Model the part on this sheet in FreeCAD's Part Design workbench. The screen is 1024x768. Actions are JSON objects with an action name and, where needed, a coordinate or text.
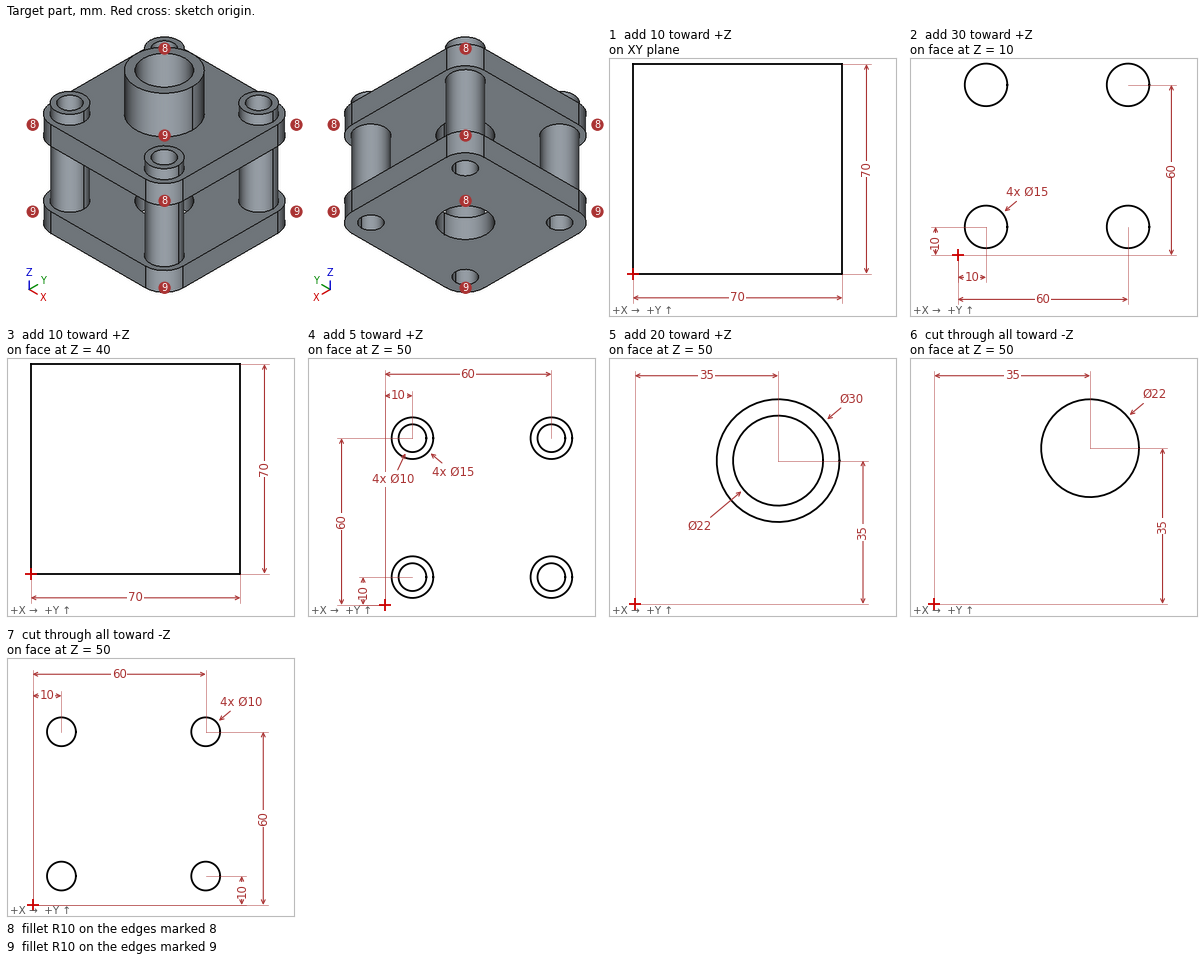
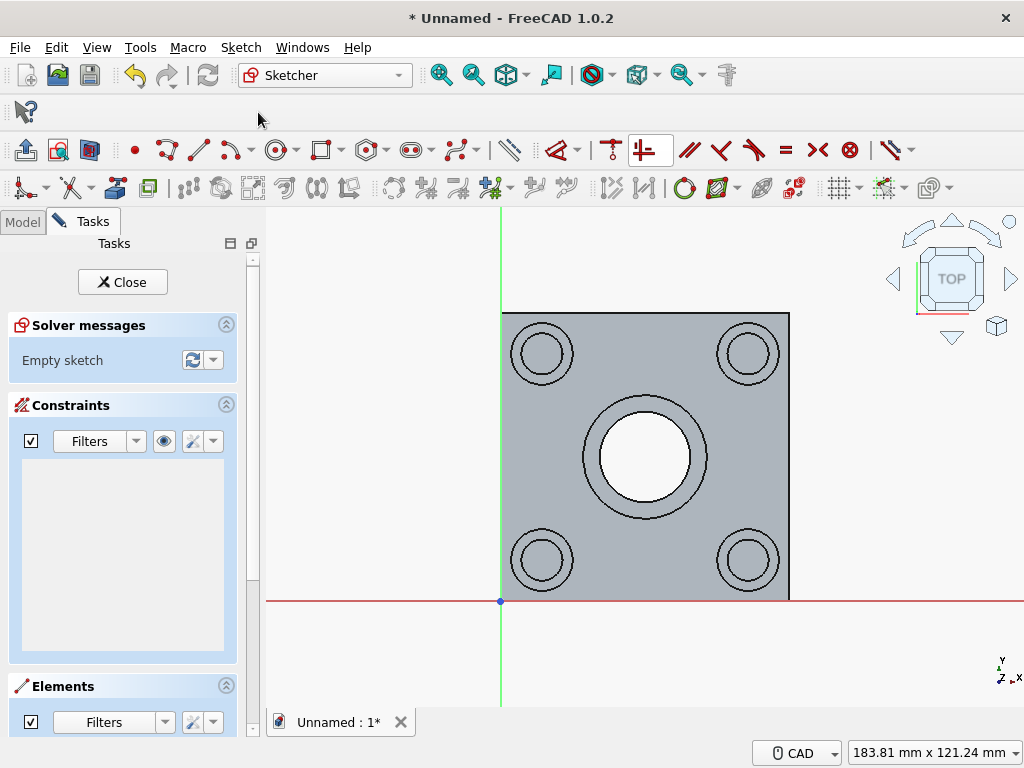
{"action": "left_click", "coordinate": [276, 150]}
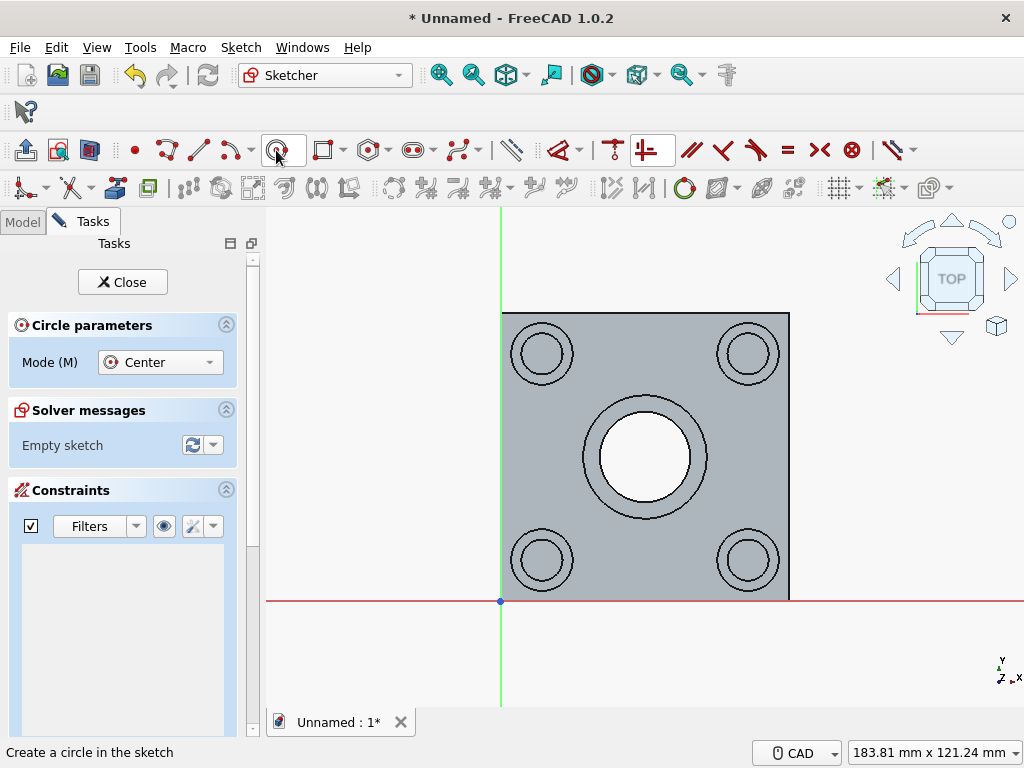
{"action": "left_click", "coordinate": [748, 354]}
{"action": "left_click", "coordinate": [763, 339]}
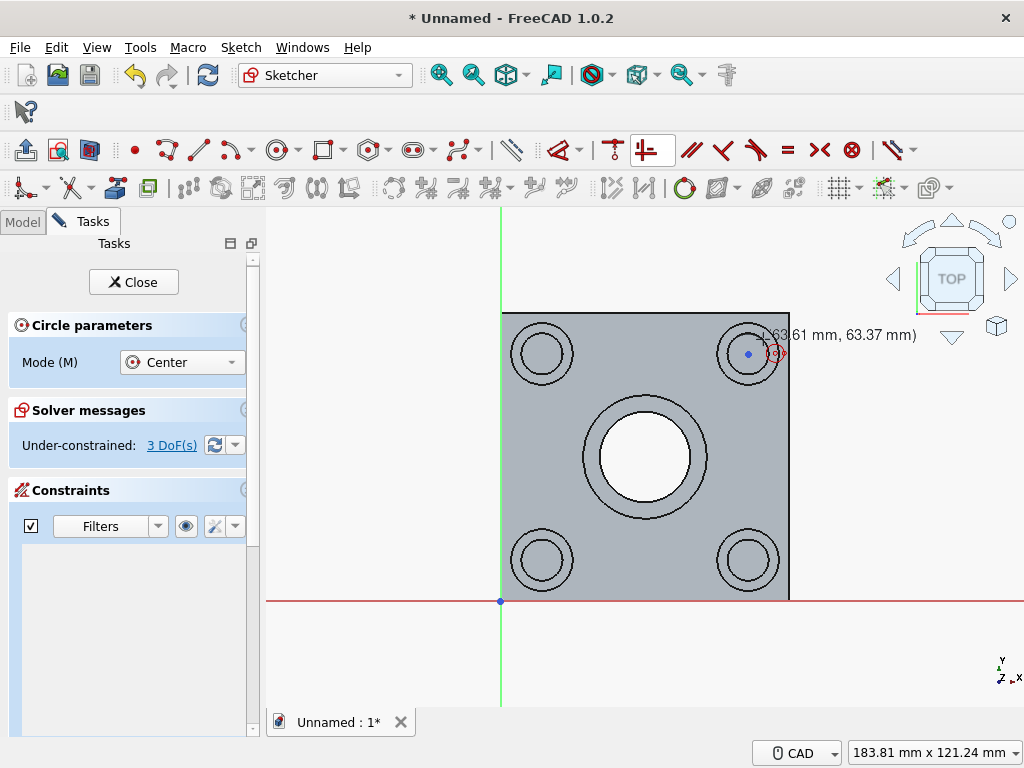
{"action": "left_click", "coordinate": [542, 354]}
{"action": "left_click", "coordinate": [556, 339]}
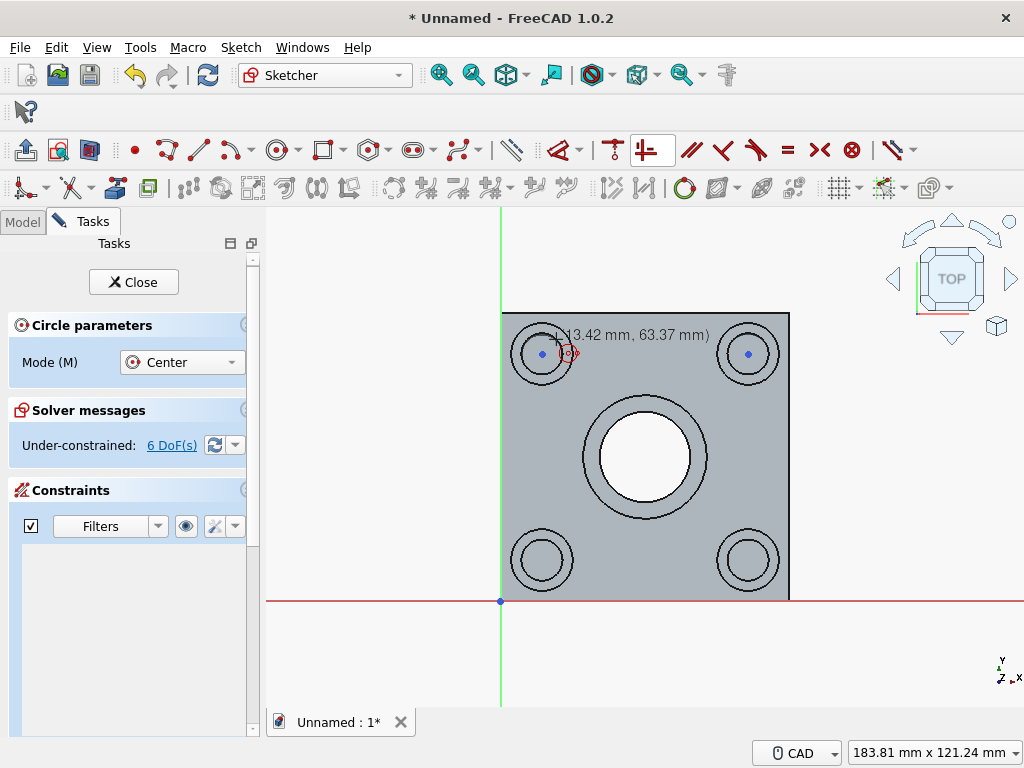
{"action": "left_click", "coordinate": [748, 560]}
{"action": "left_click", "coordinate": [763, 546]}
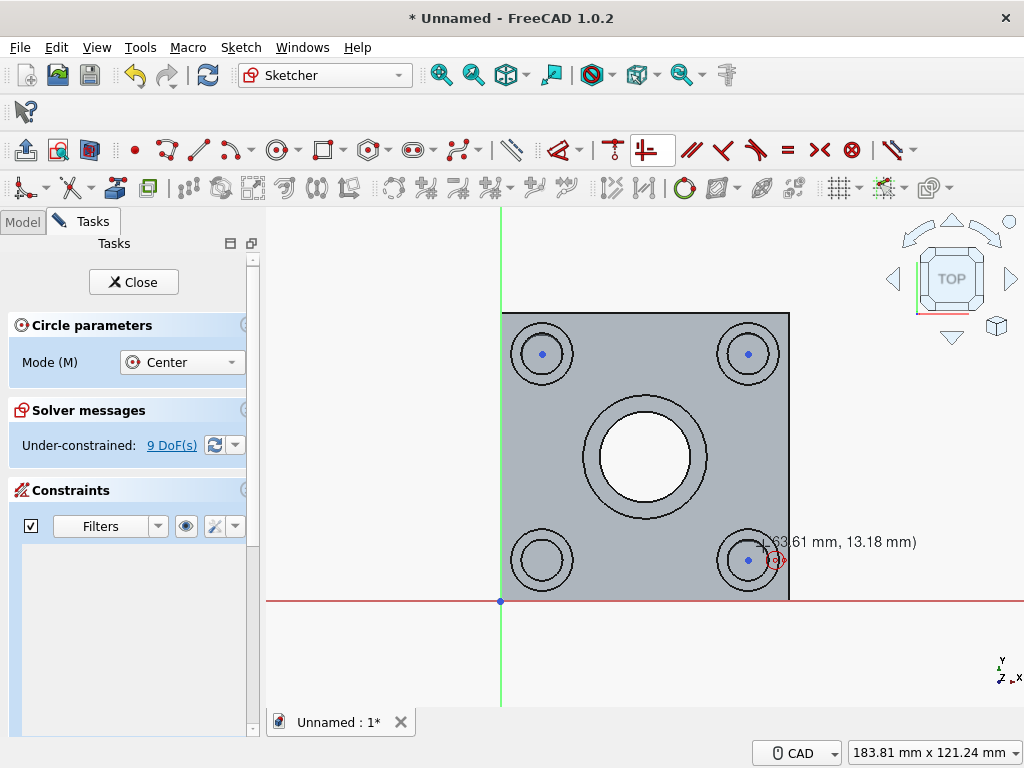
{"action": "left_click", "coordinate": [542, 560]}
{"action": "left_click", "coordinate": [556, 546]}
{"action": "key", "text": "Escape"}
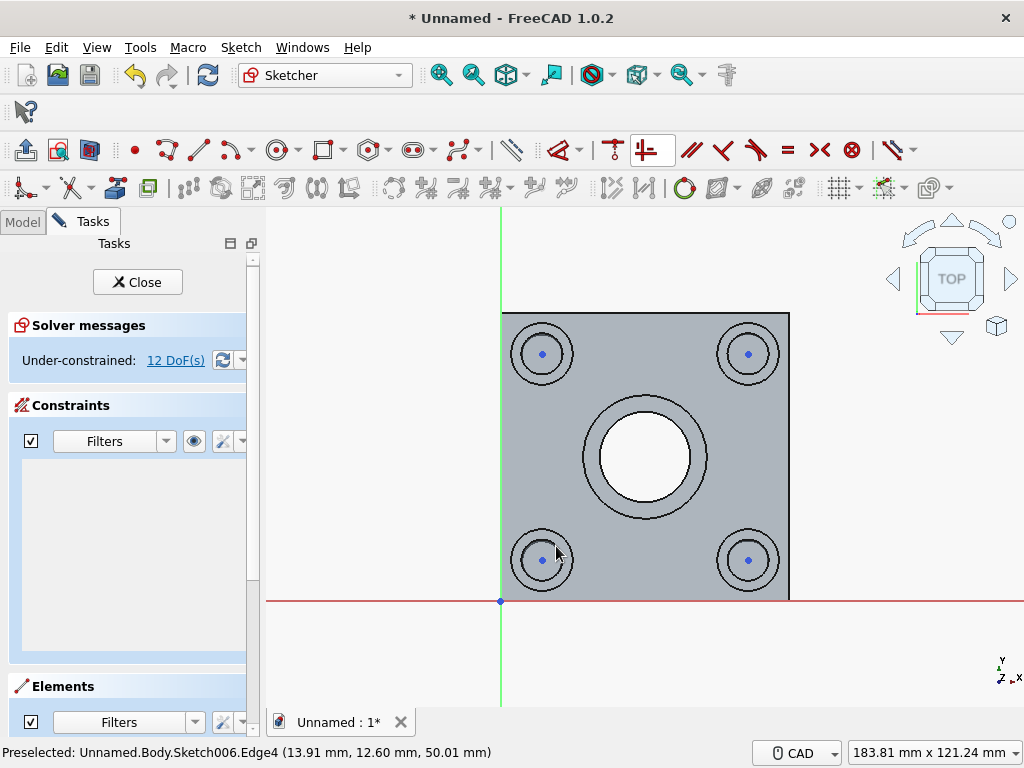
{"action": "left_click", "coordinate": [763, 340]}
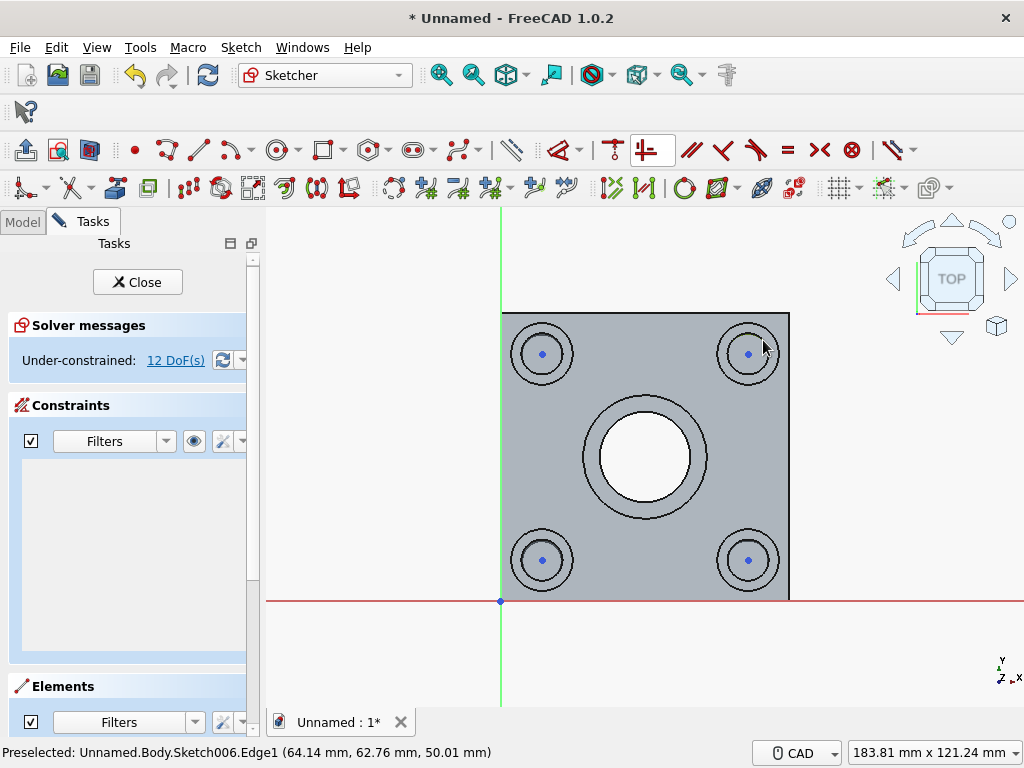
{"action": "left_click", "coordinate": [556, 340]}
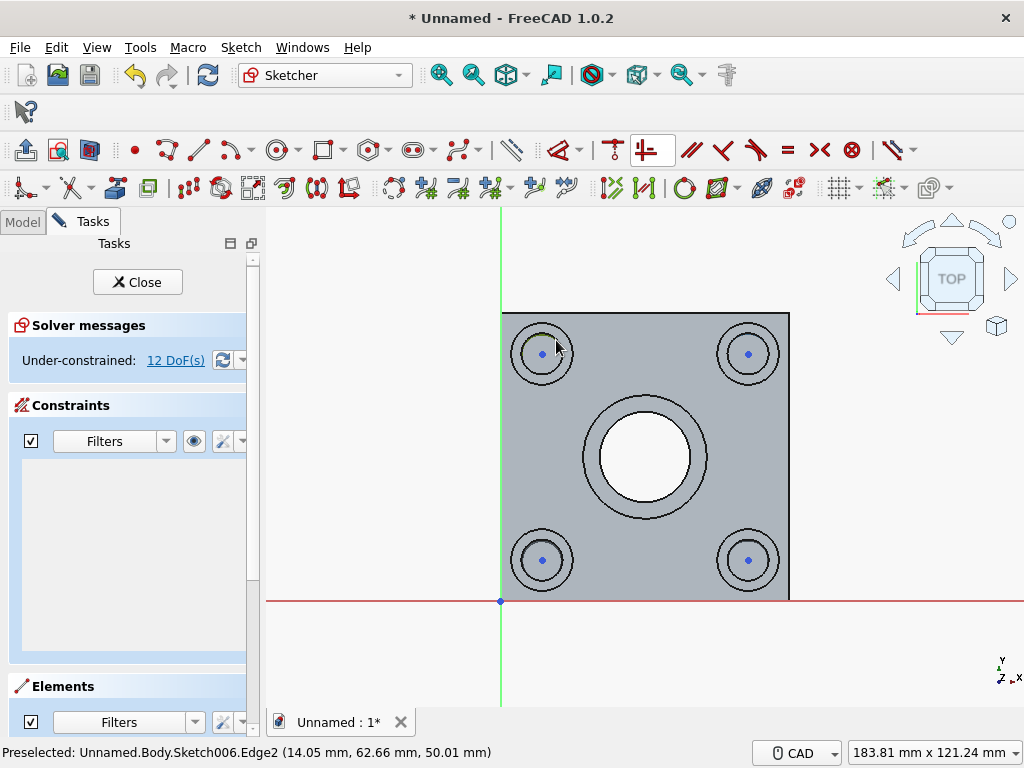
{"action": "left_click", "coordinate": [762, 546]}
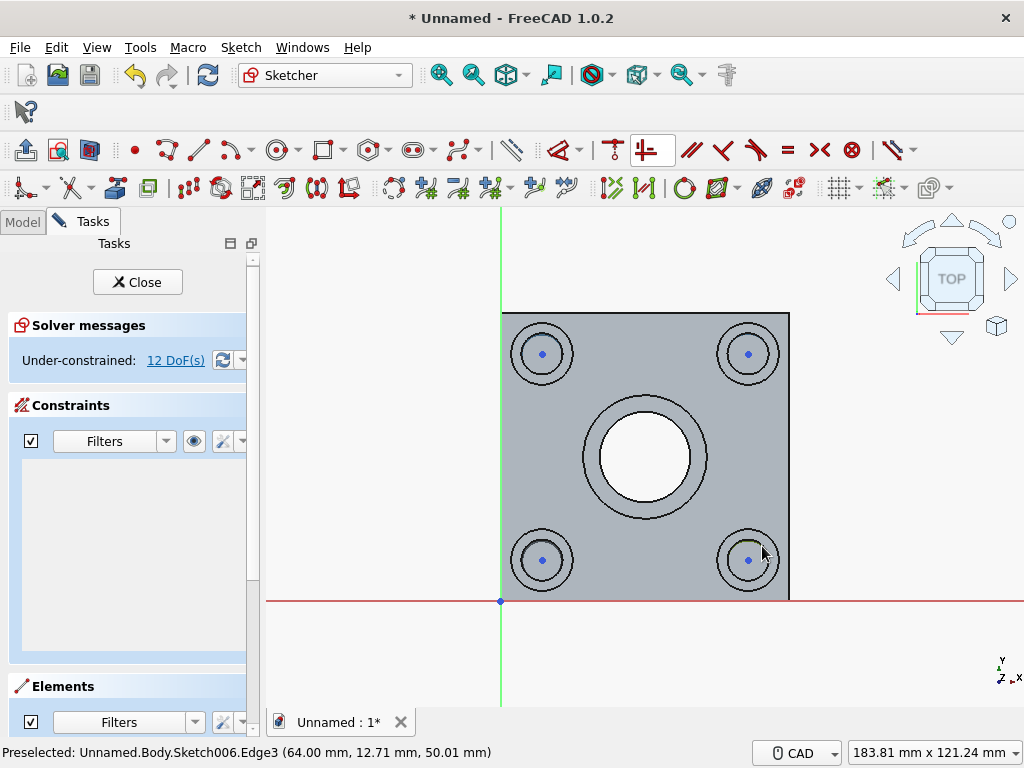
{"action": "left_click", "coordinate": [556, 547]}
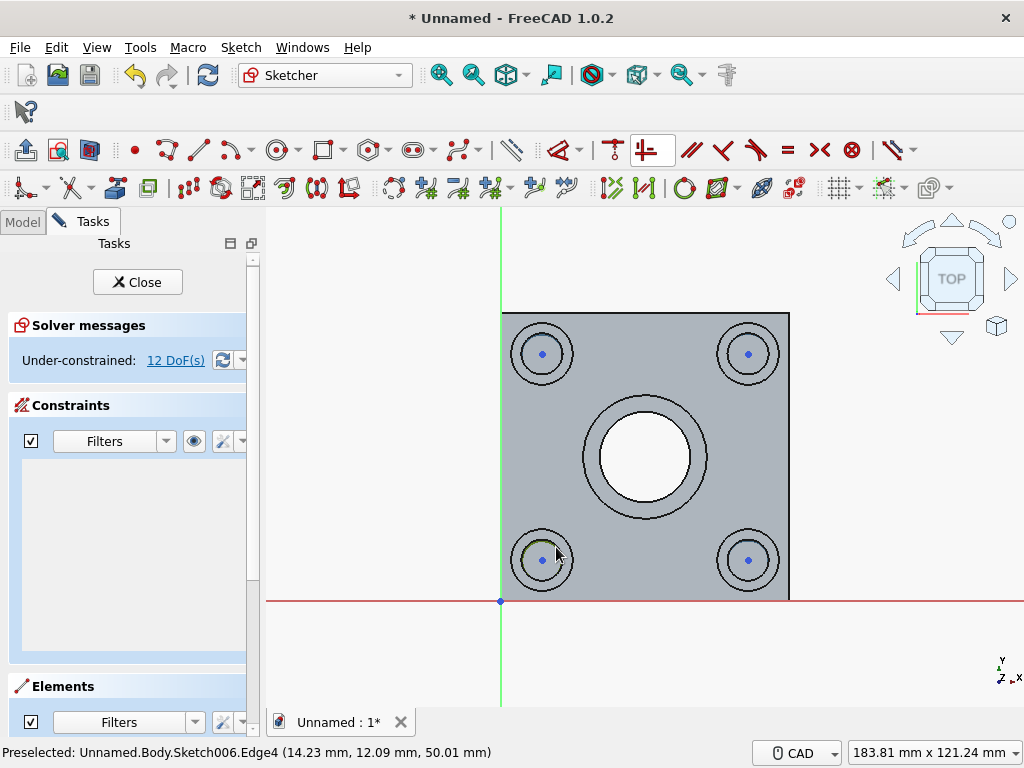
{"action": "left_click", "coordinate": [788, 150]}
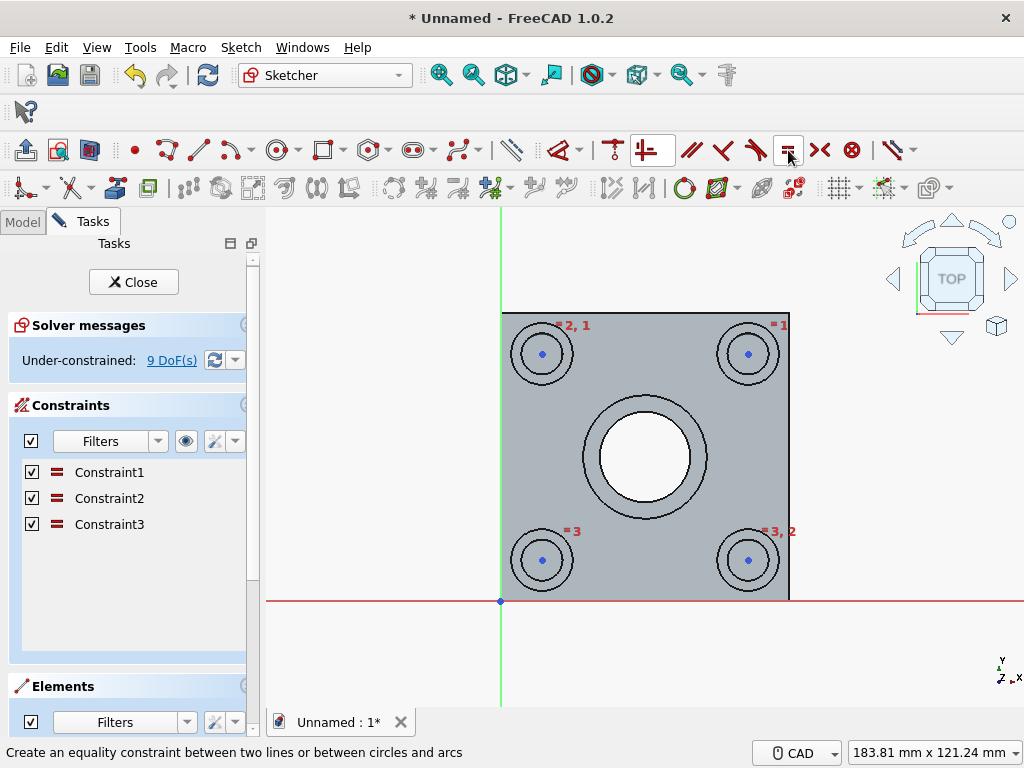
{"action": "left_click", "coordinate": [748, 355]}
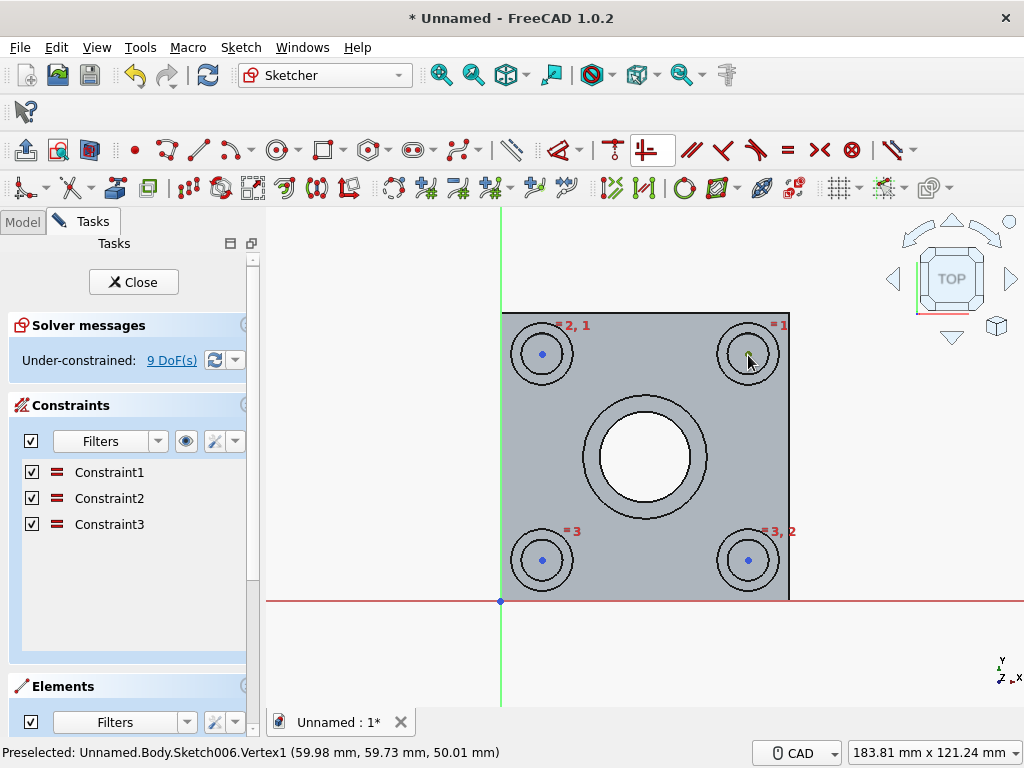
{"action": "left_click", "coordinate": [542, 355]}